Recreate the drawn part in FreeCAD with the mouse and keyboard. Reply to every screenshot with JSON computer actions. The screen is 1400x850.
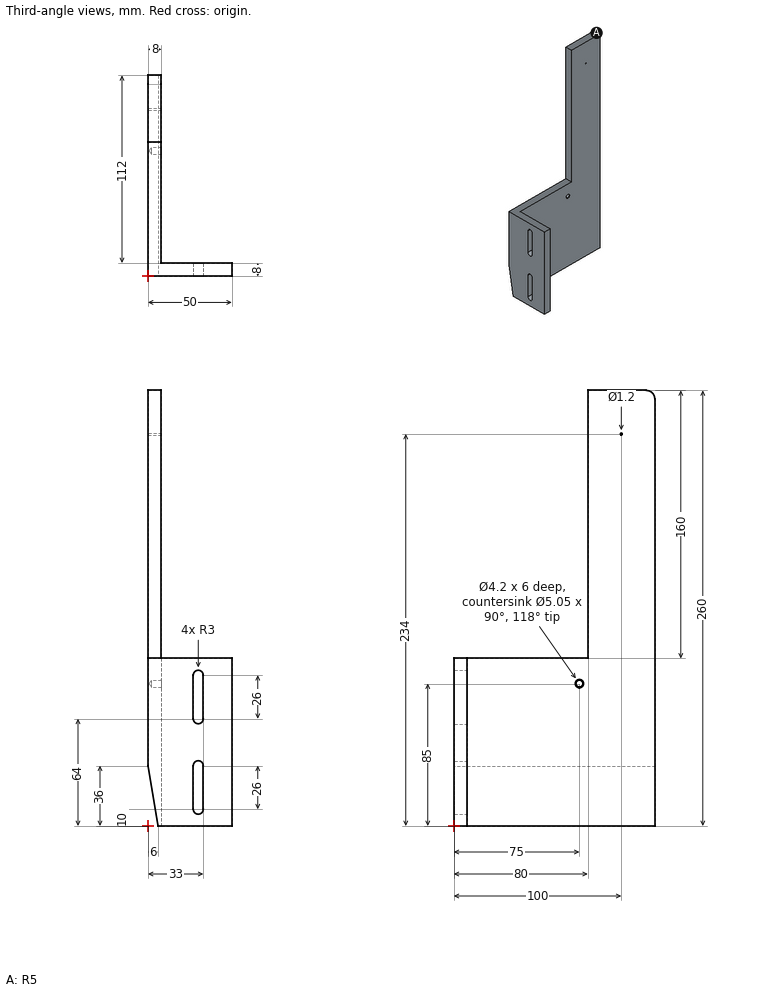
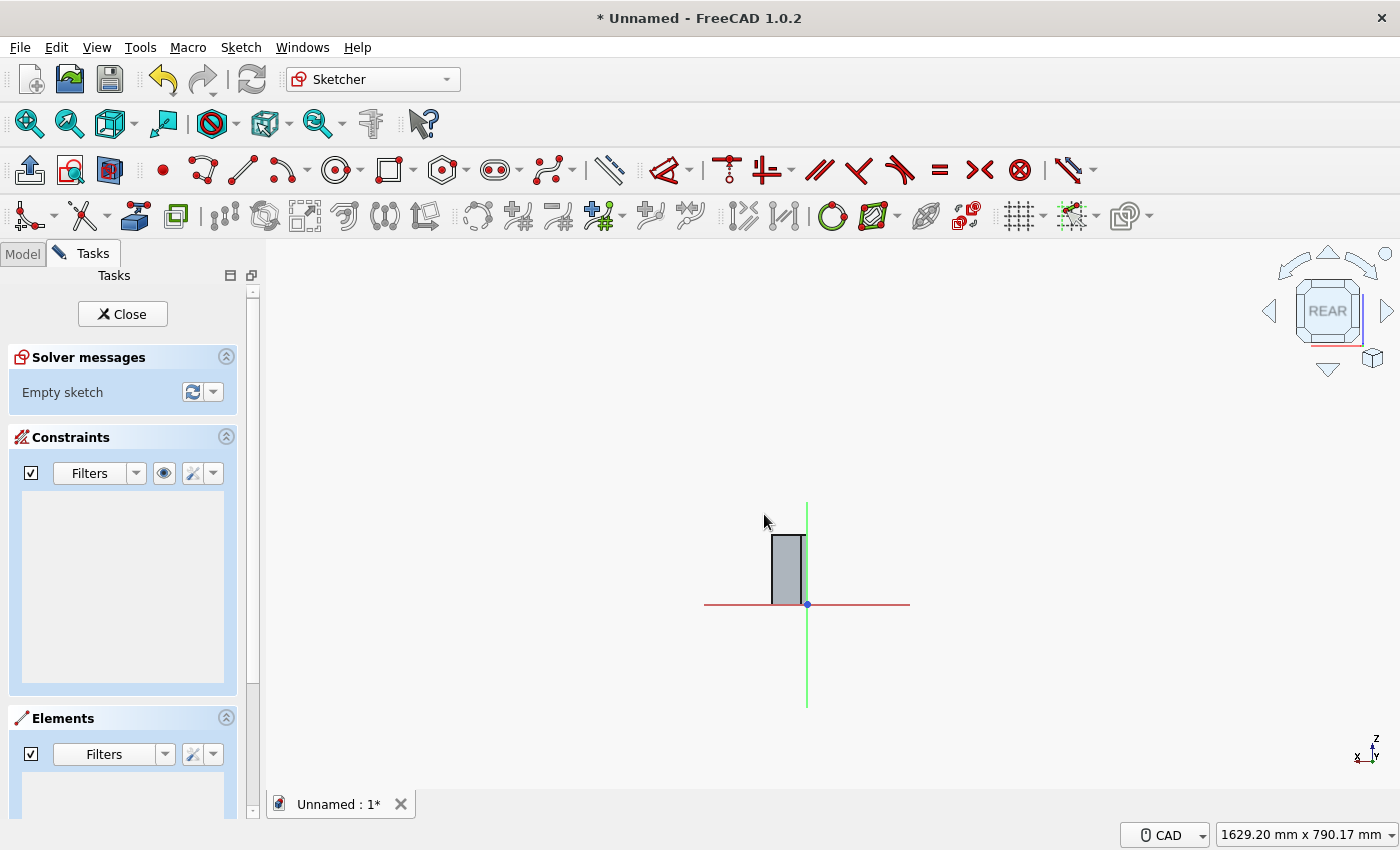
{"action": "scroll", "coordinate": [803, 587], "scroll_direction": "up", "scroll_amount": 8}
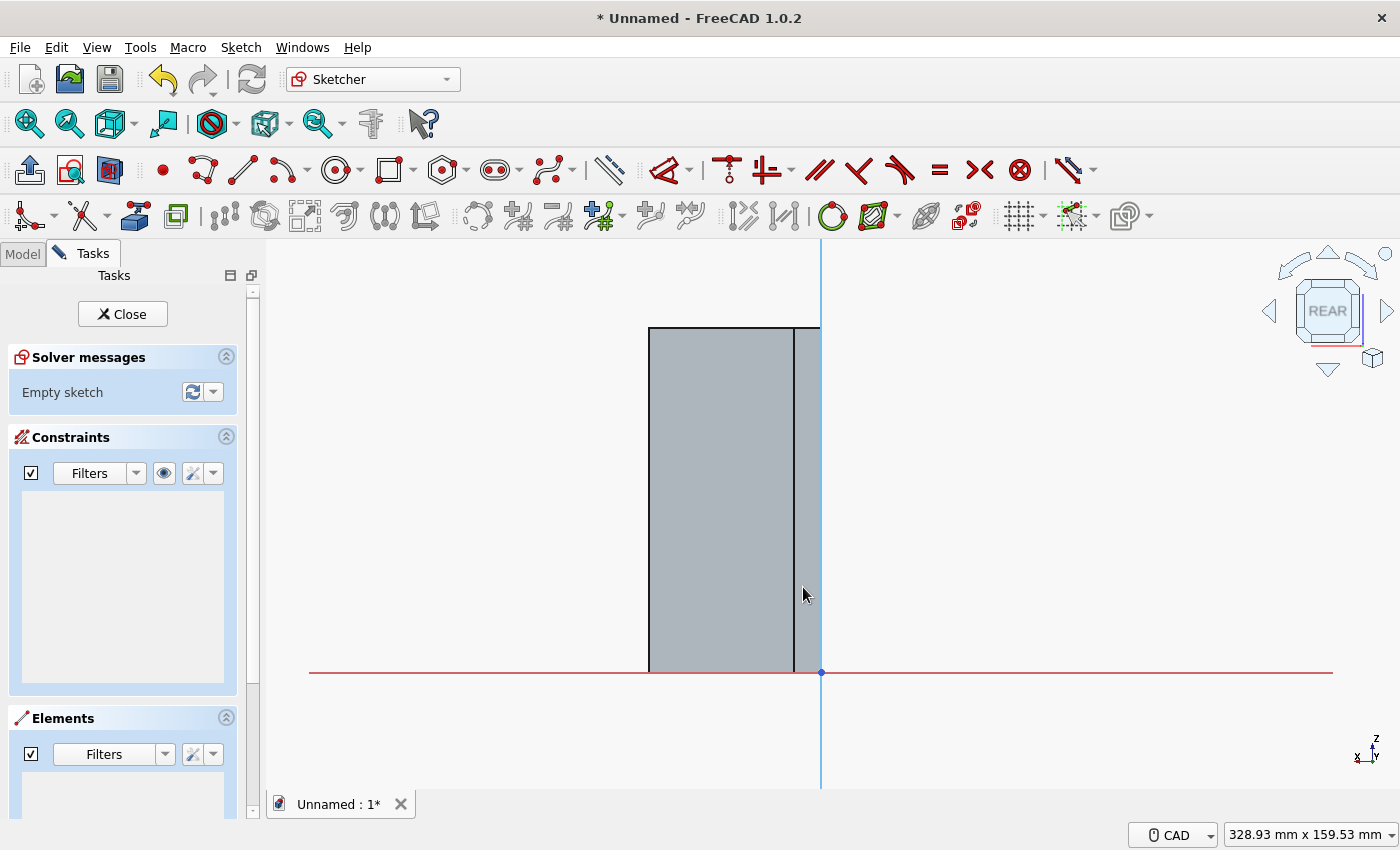
{"action": "left_click", "coordinate": [496, 170]}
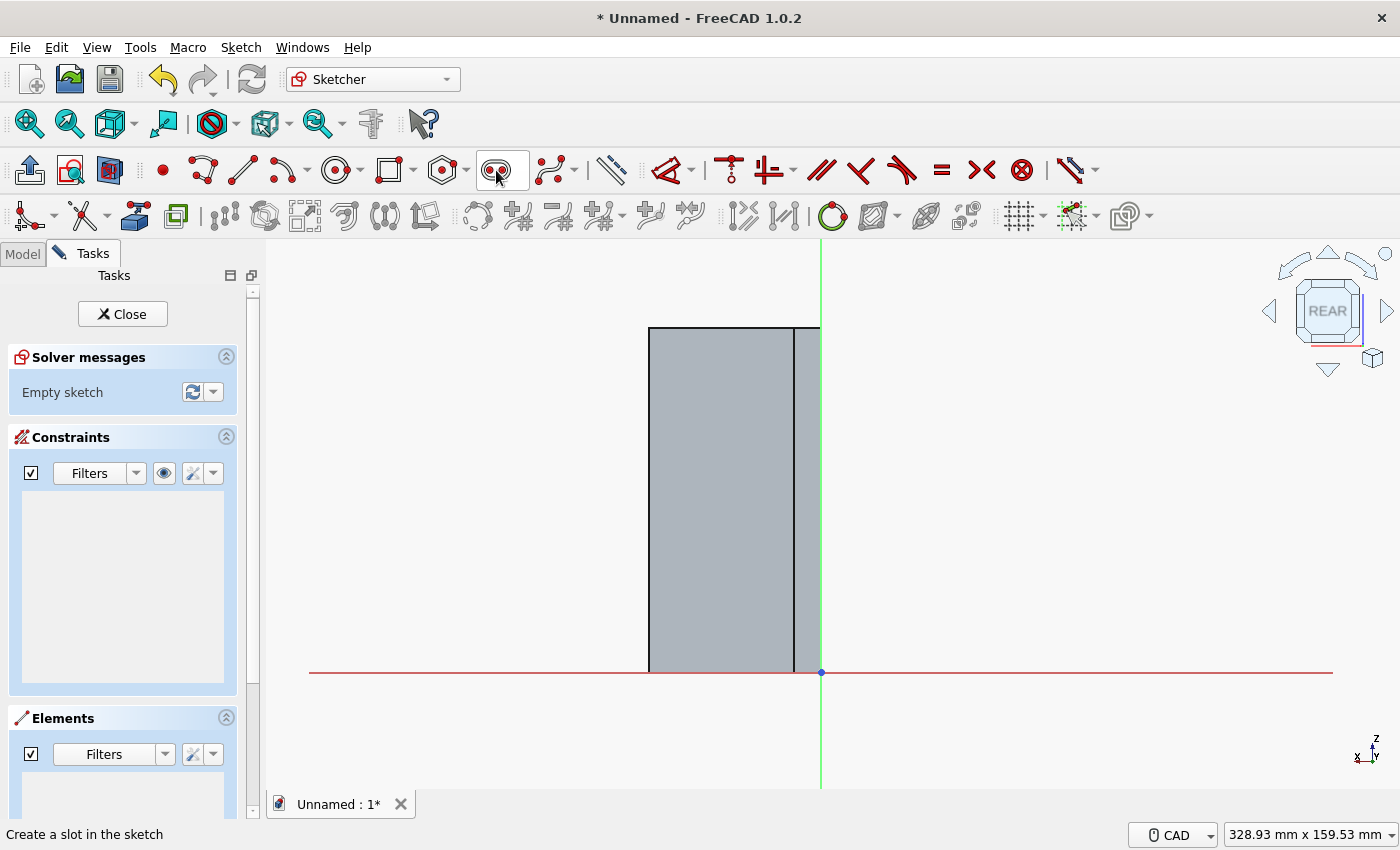
{"action": "scroll", "coordinate": [718, 452], "scroll_direction": "up", "scroll_amount": 4}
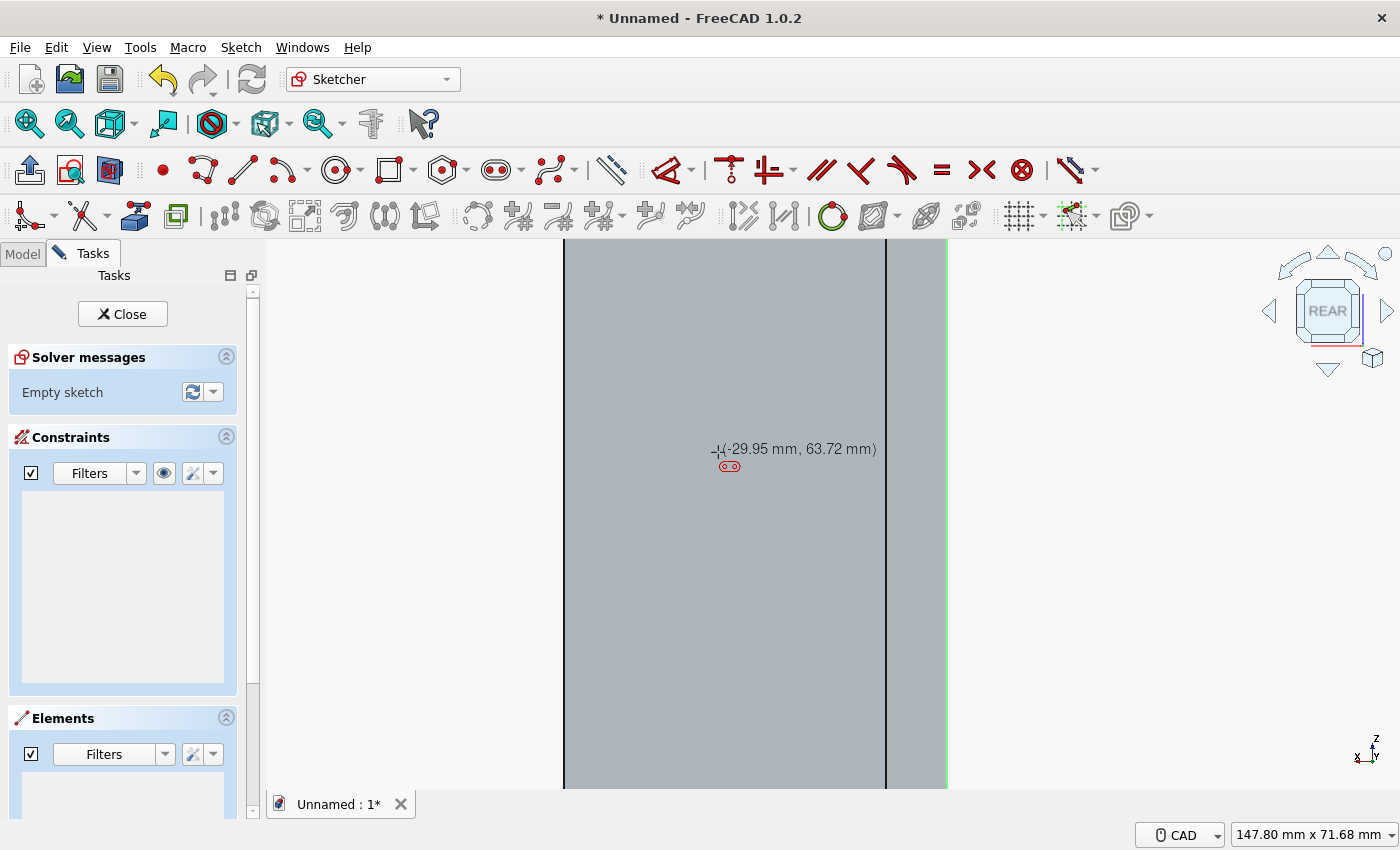
{"action": "left_click", "coordinate": [717, 452]}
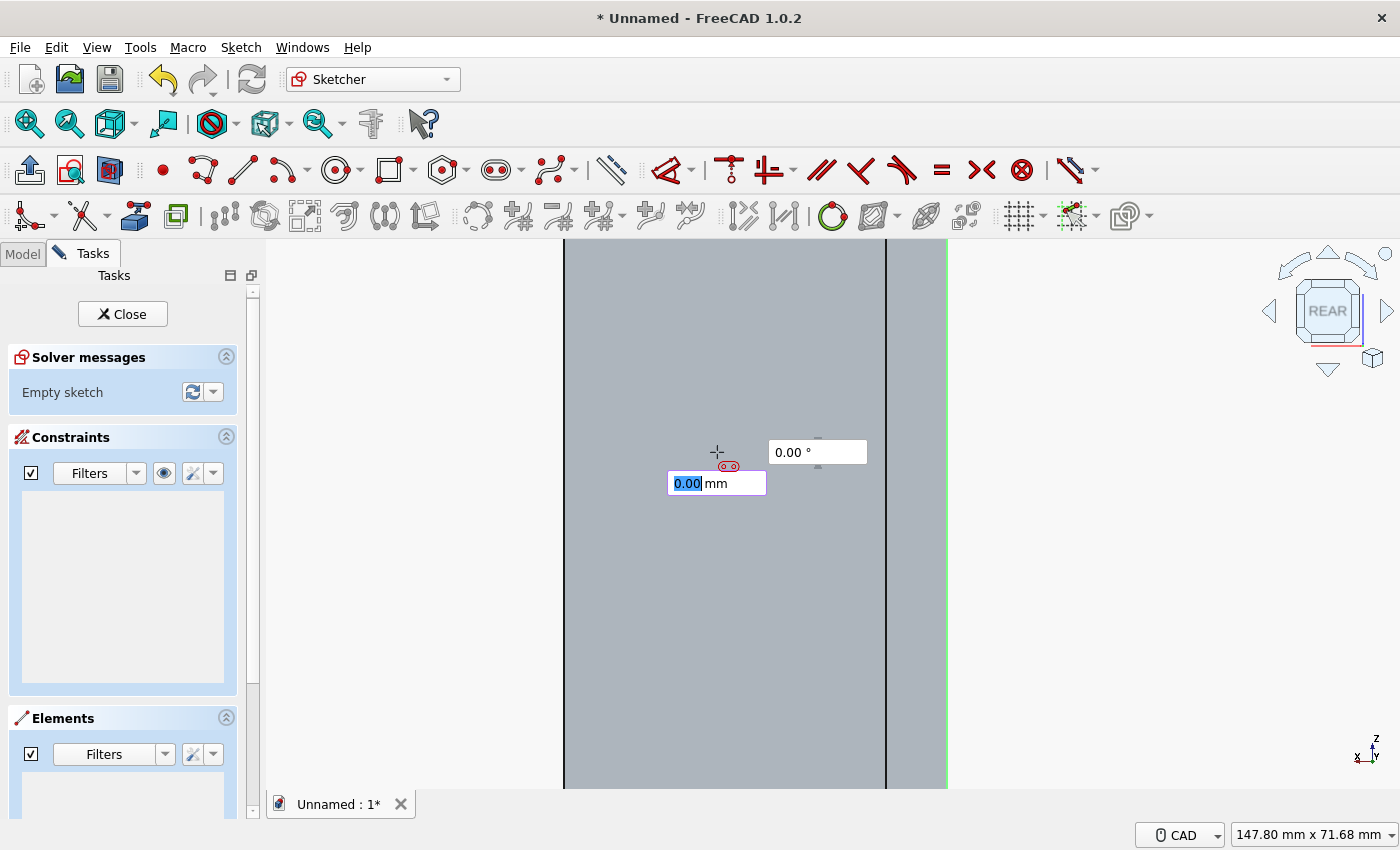
{"action": "scroll", "coordinate": [719, 455], "scroll_direction": "down", "scroll_amount": 4}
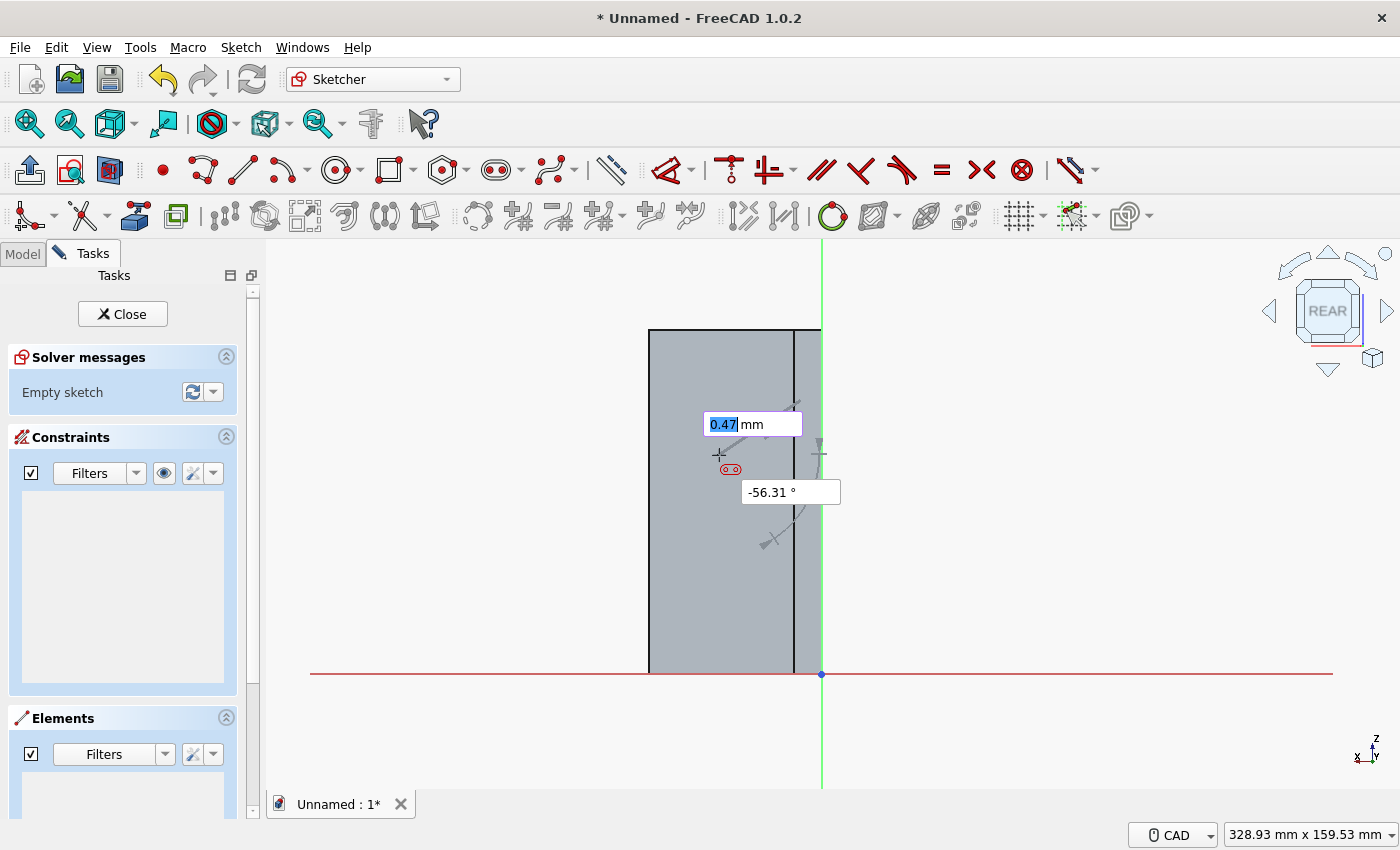
{"action": "left_click", "coordinate": [718, 364]}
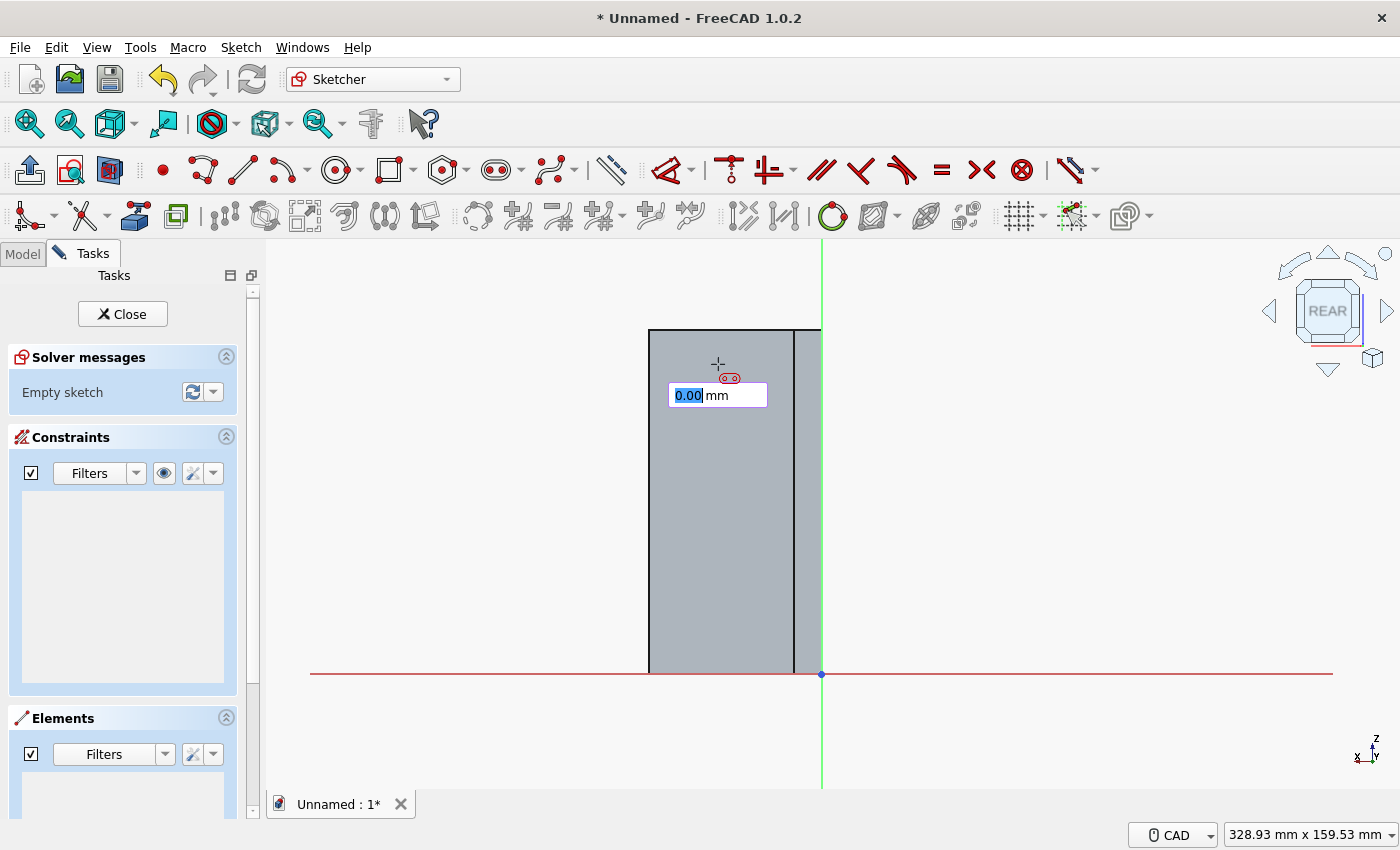
{"action": "scroll", "coordinate": [729, 409], "scroll_direction": "up", "scroll_amount": 3}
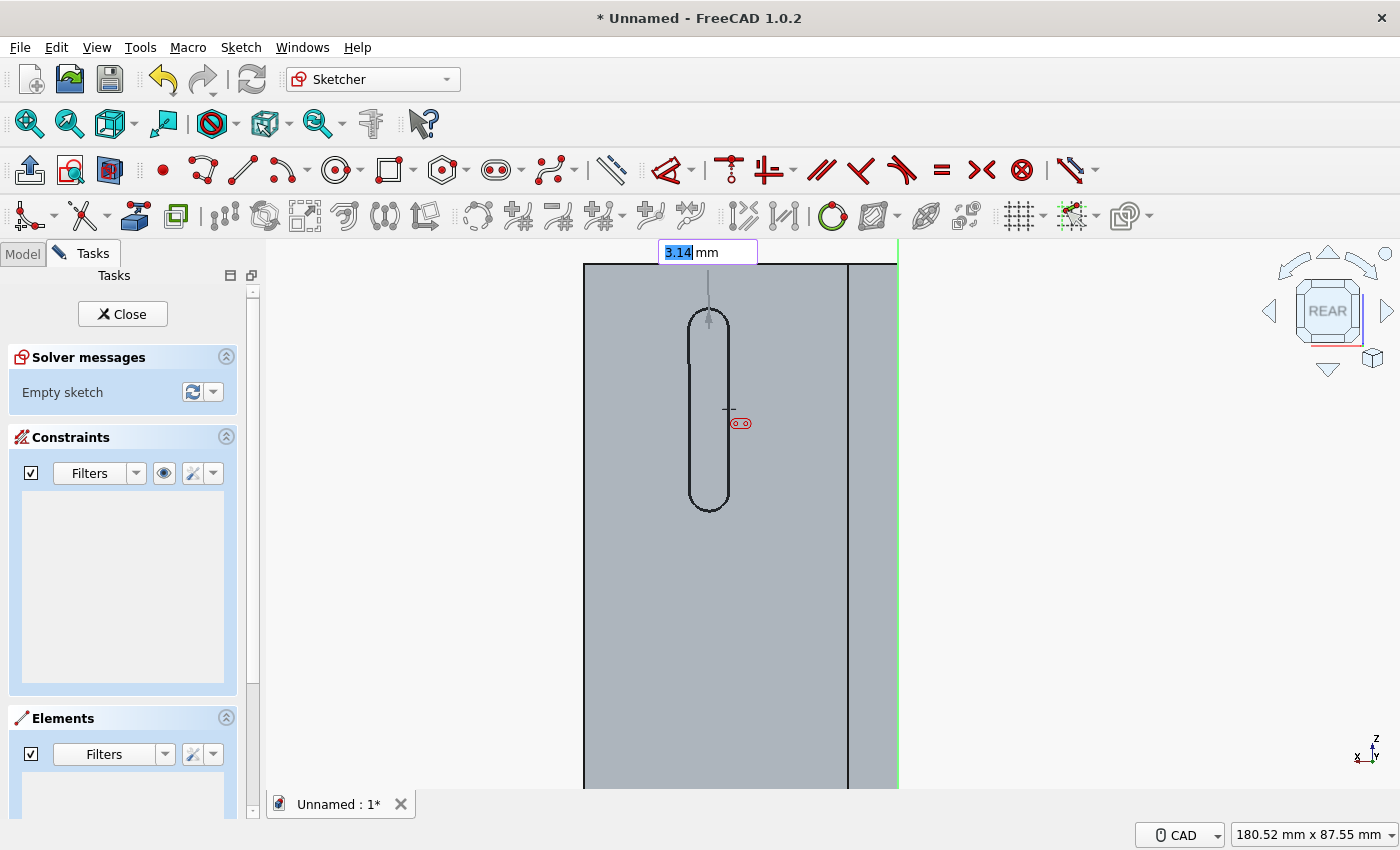
{"action": "left_click", "coordinate": [728, 409]}